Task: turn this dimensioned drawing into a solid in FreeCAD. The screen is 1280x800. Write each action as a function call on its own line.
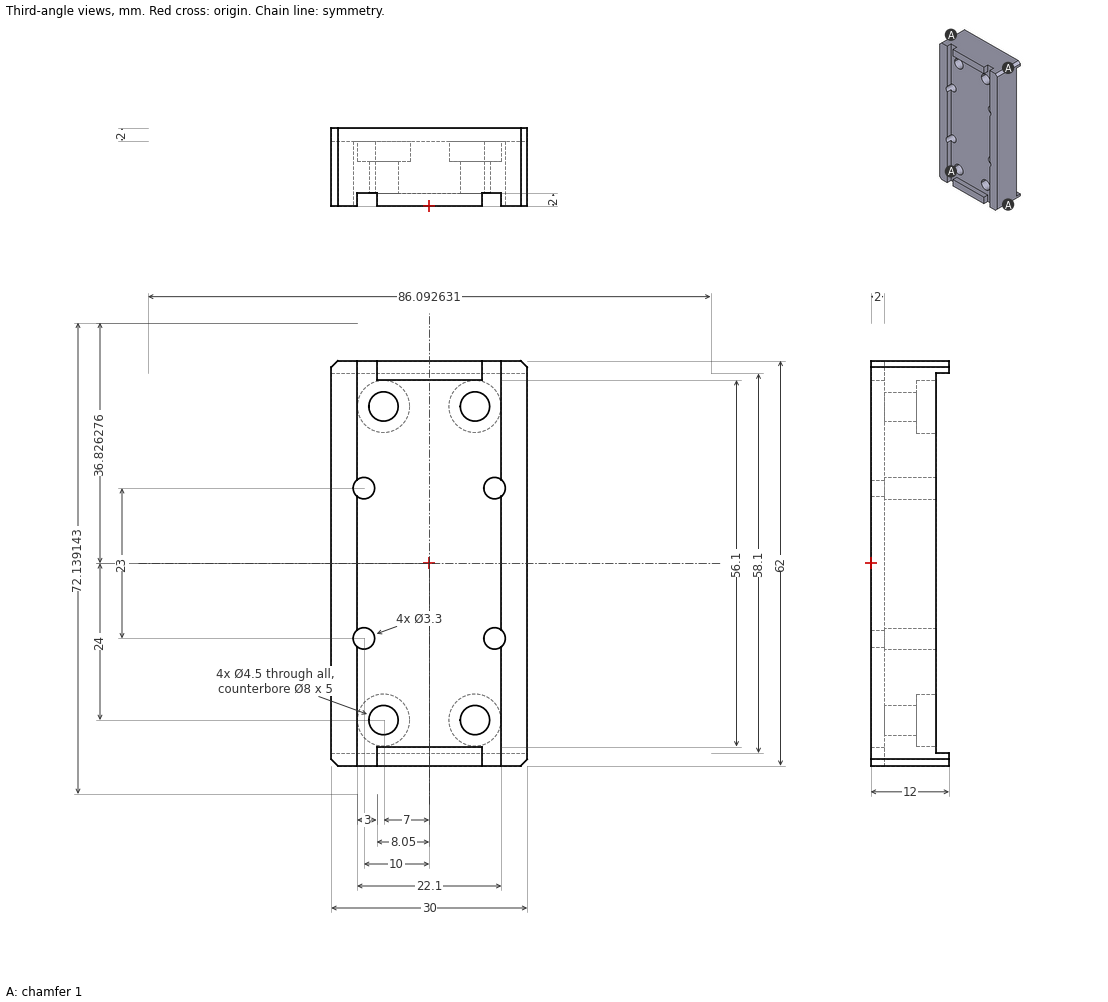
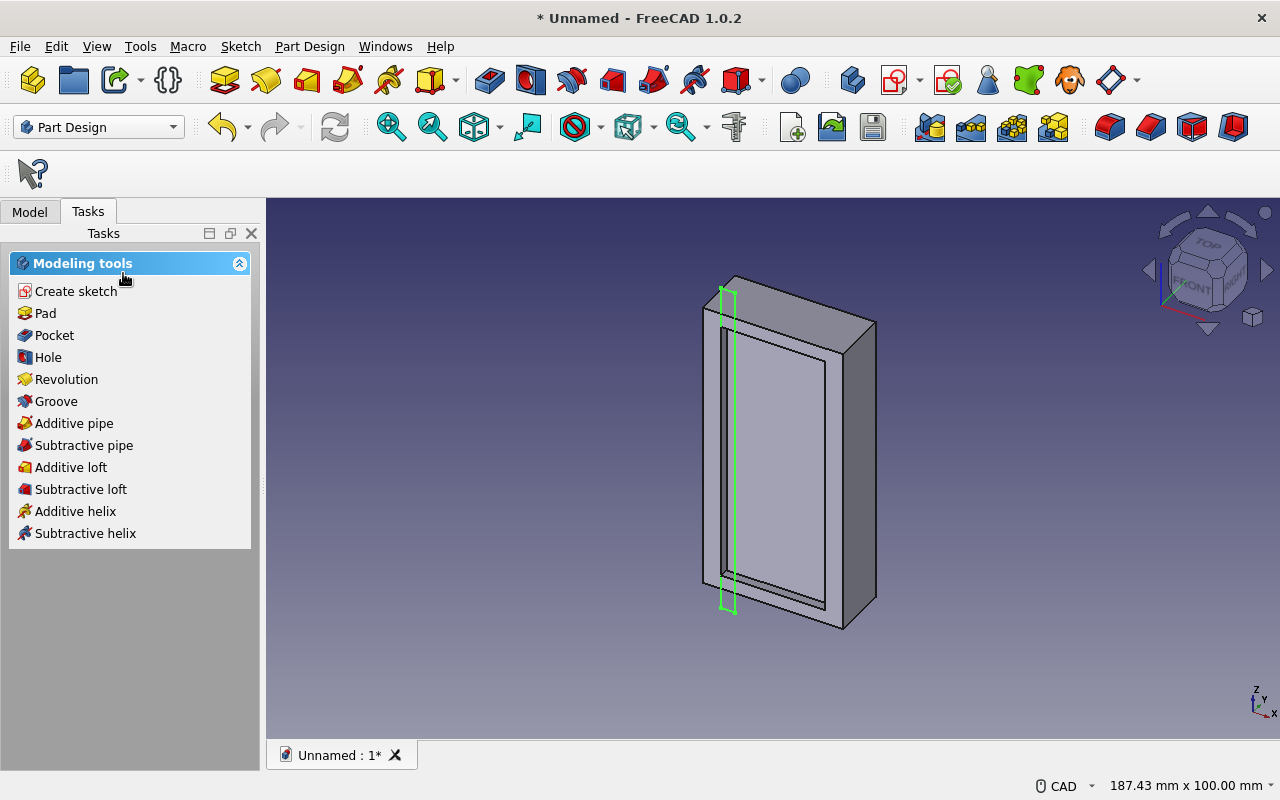
click(490, 80)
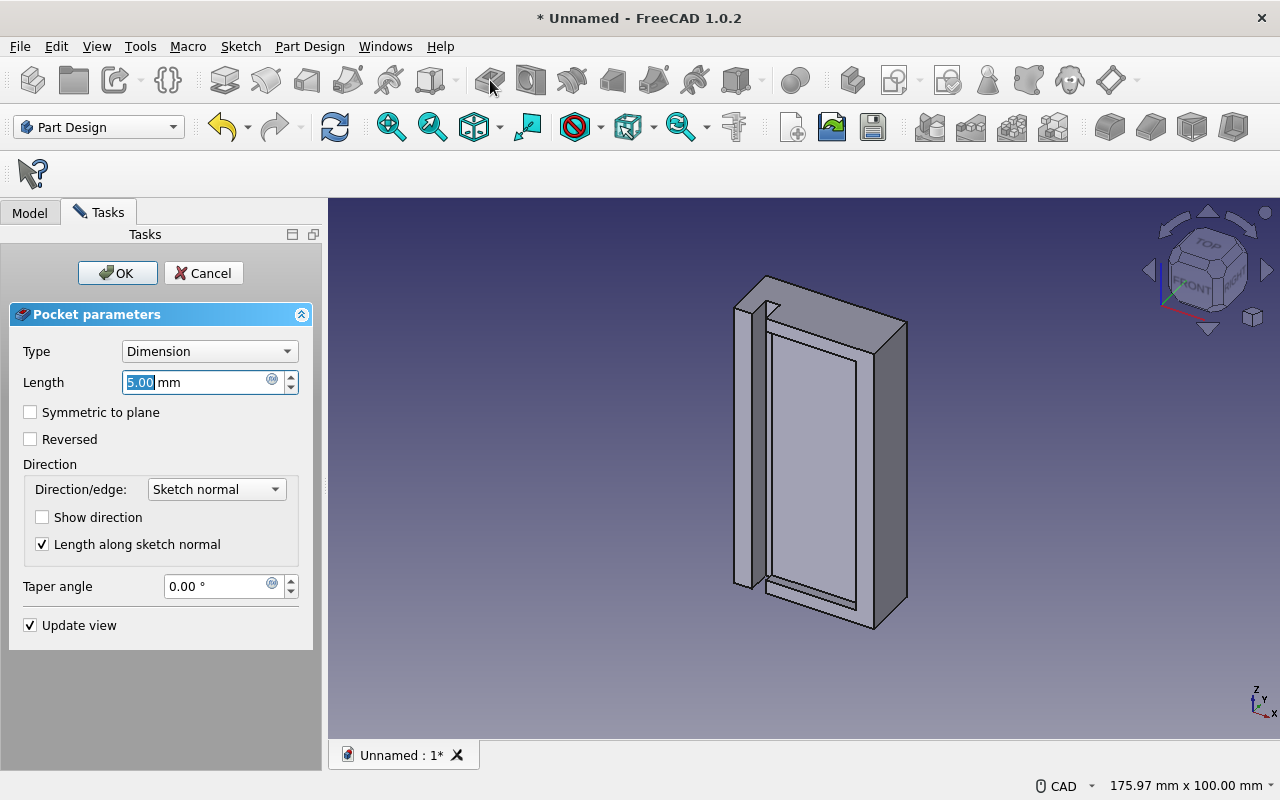
text(2)
key(Tab)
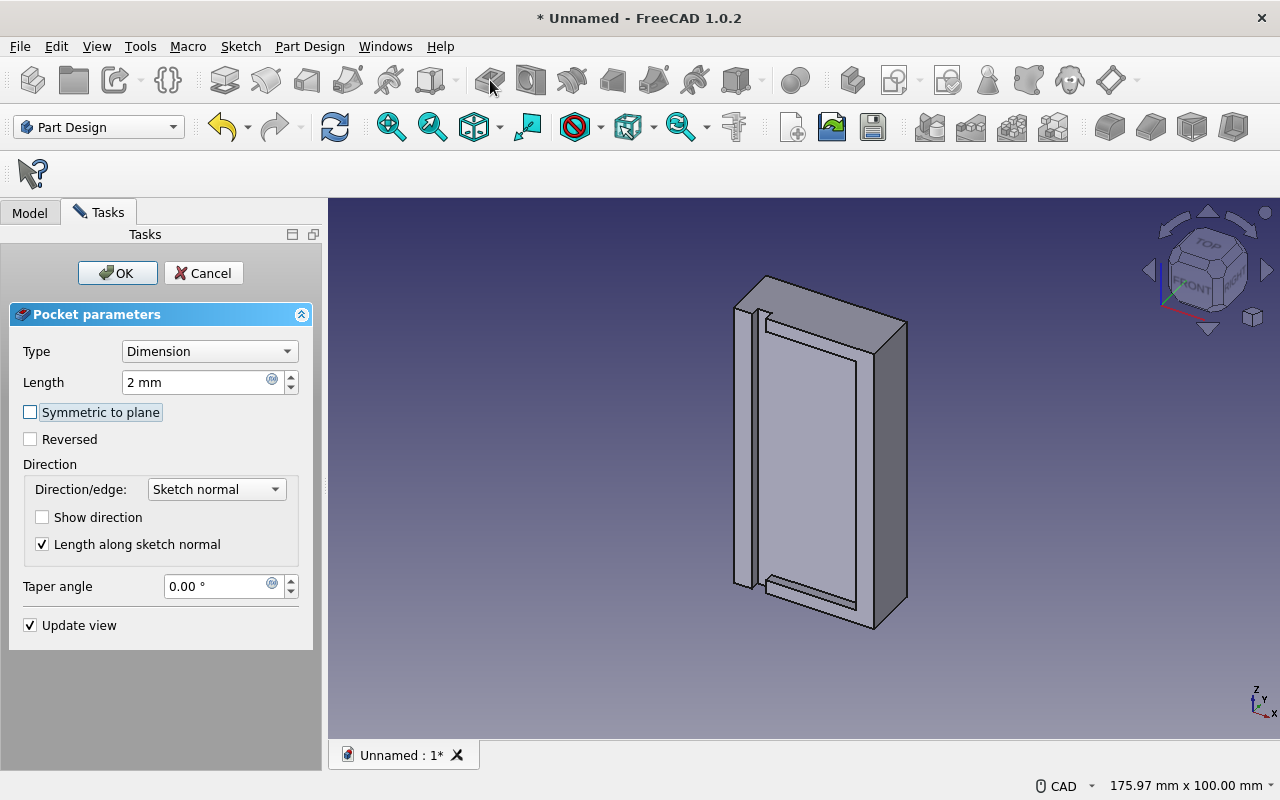
click(118, 273)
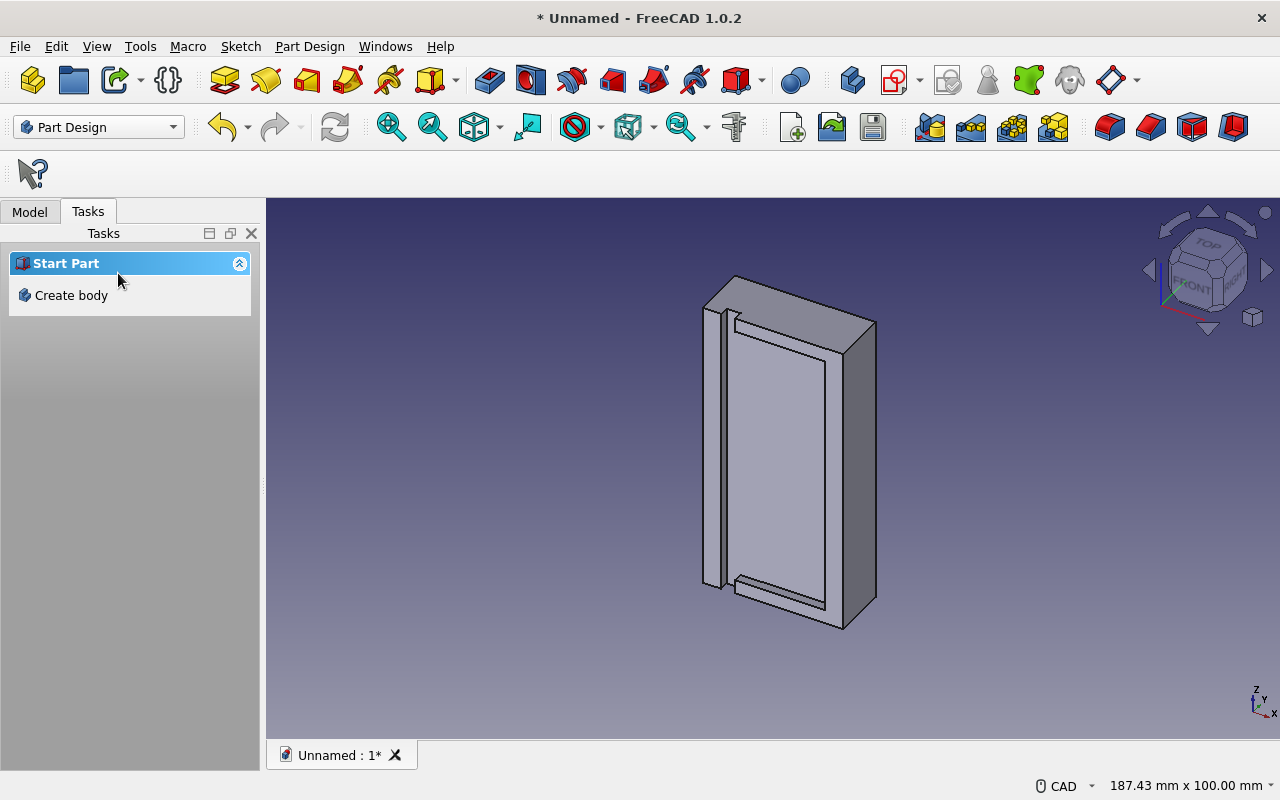
click(30, 212)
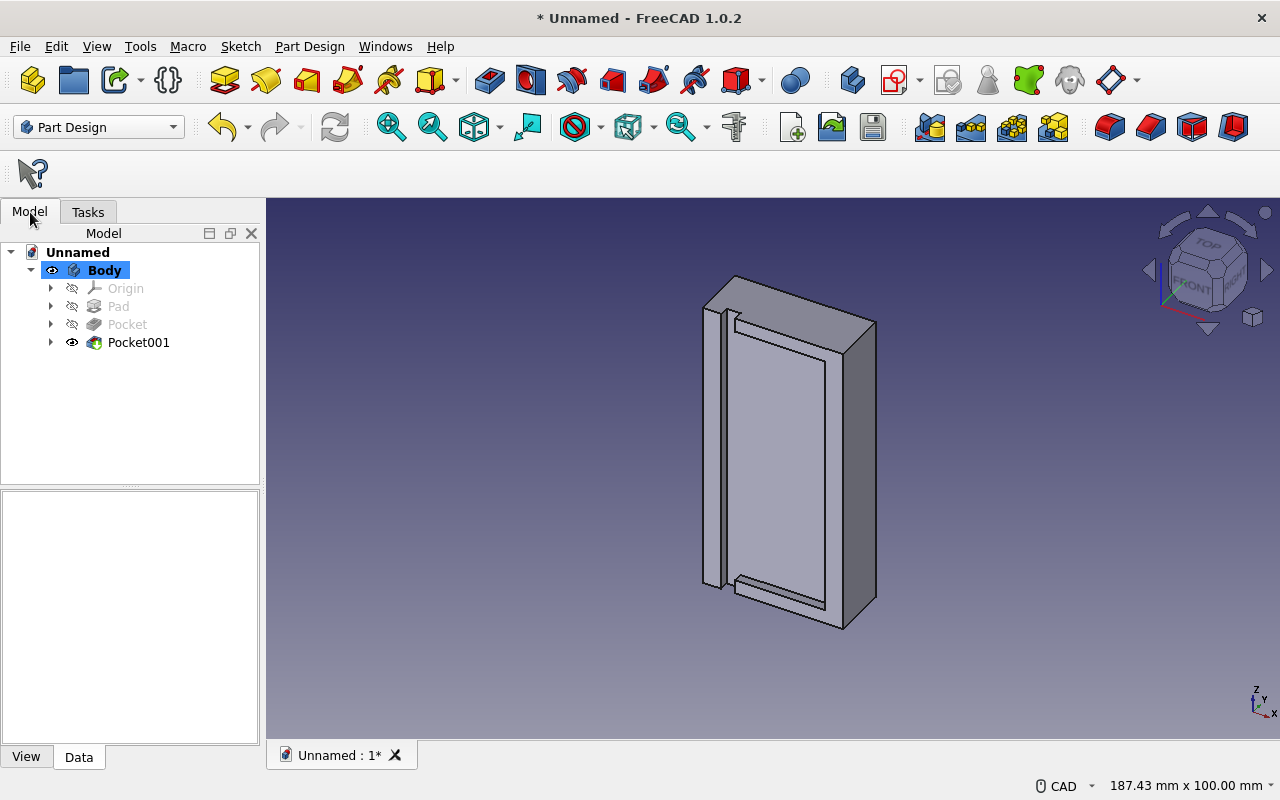
click(117, 342)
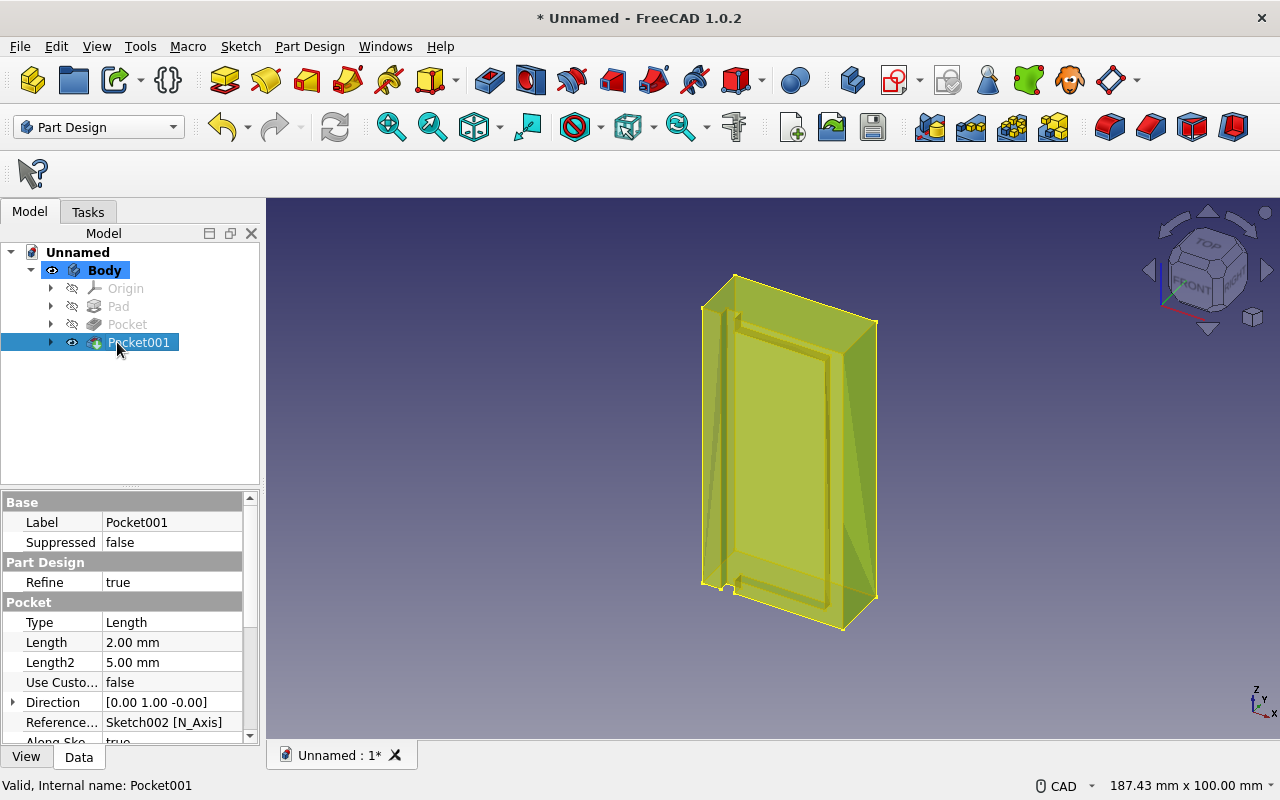
click(930, 128)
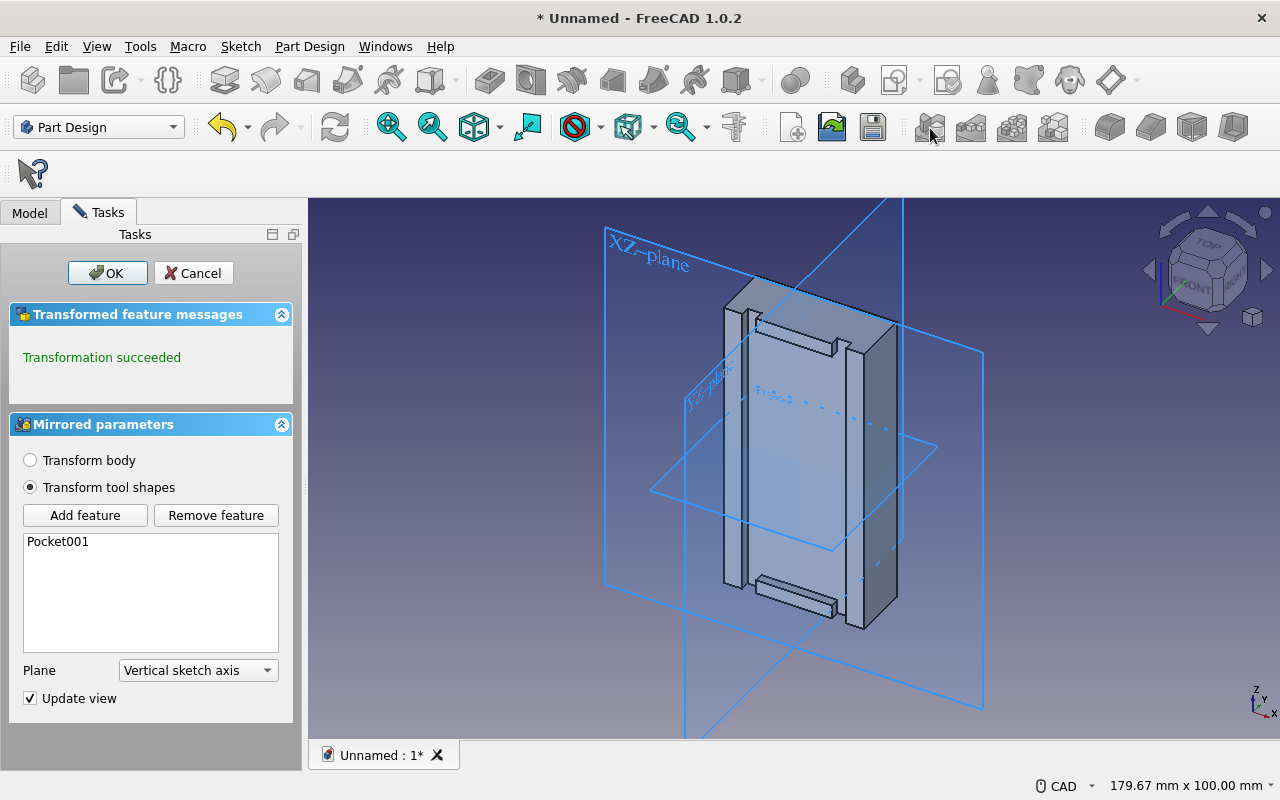
click(199, 670)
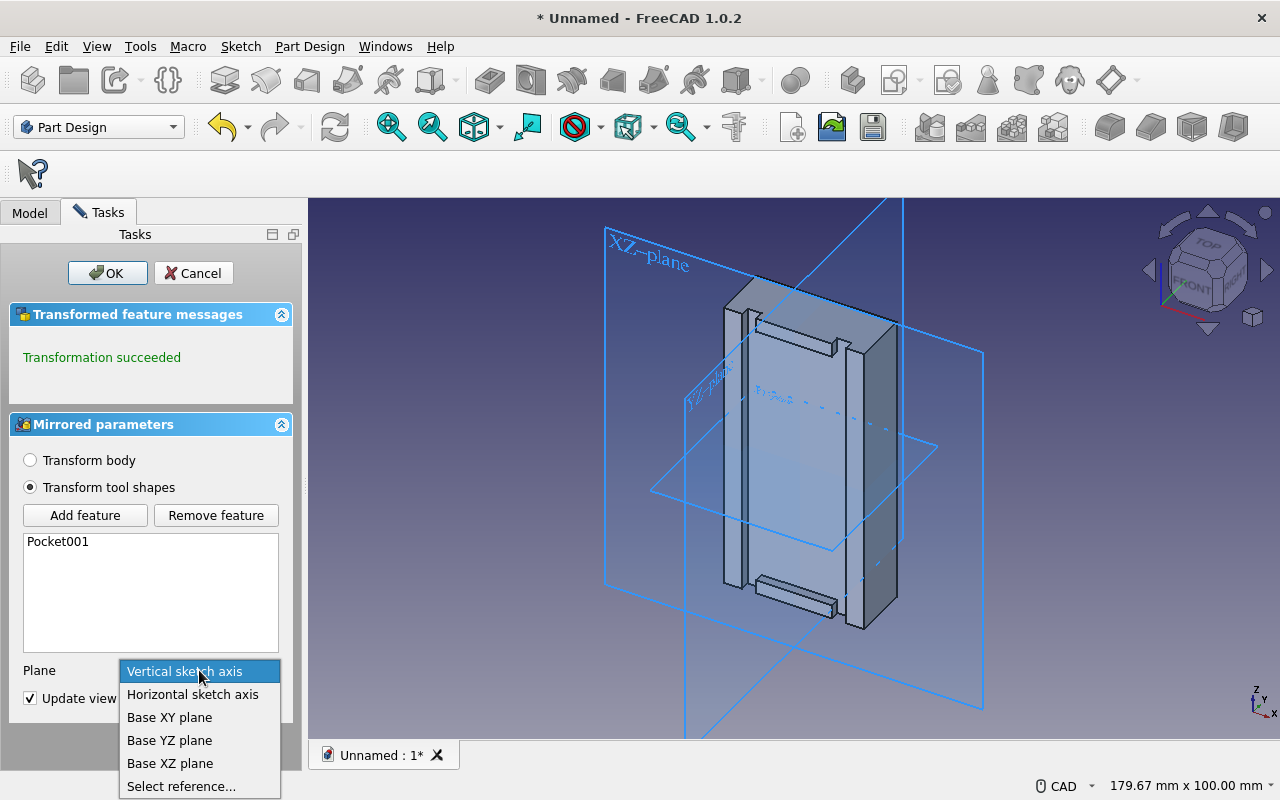
click(198, 740)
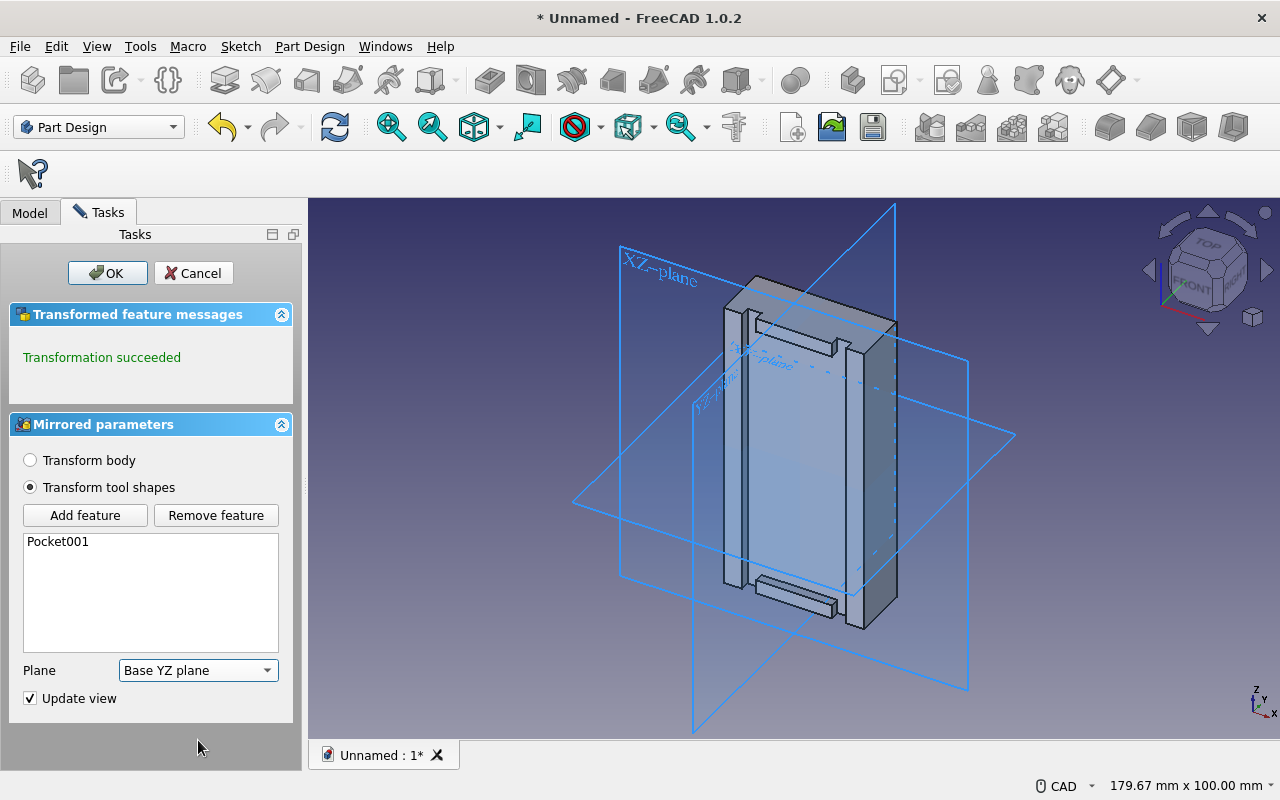
click(108, 273)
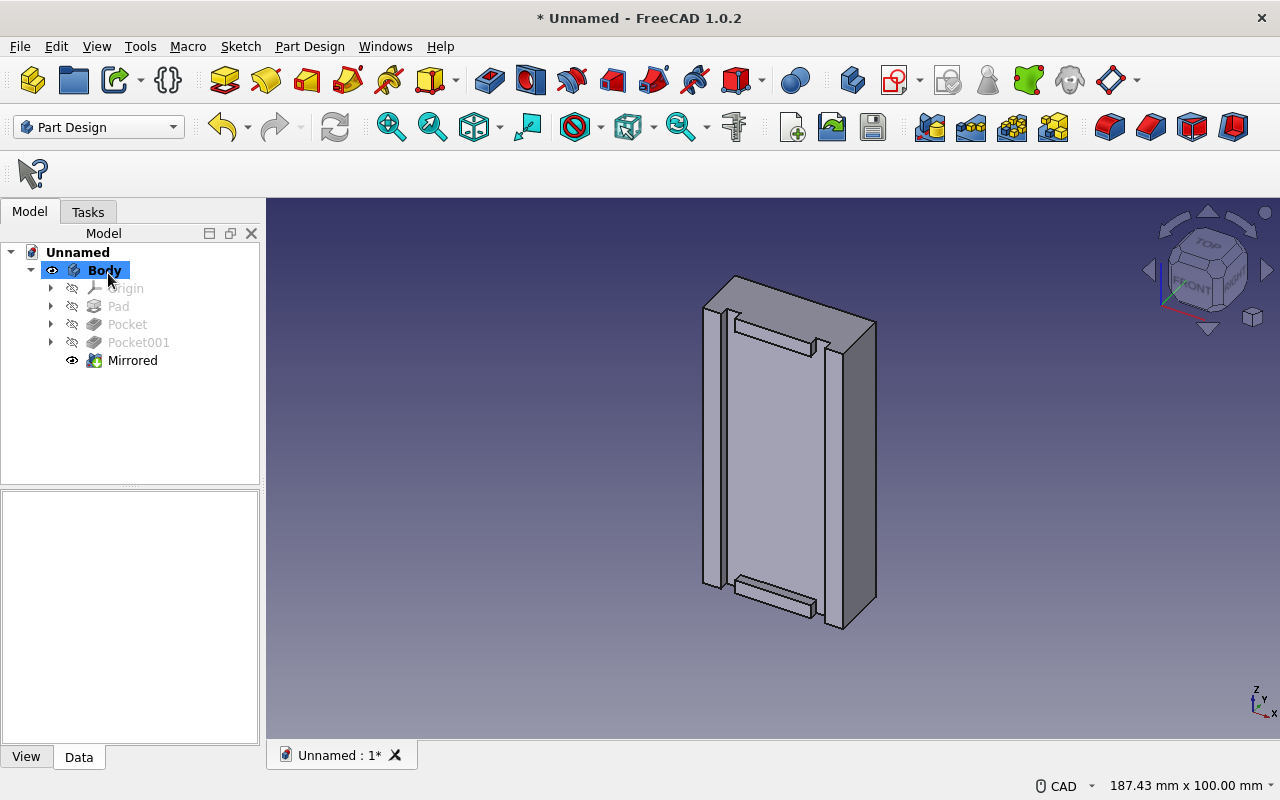
key(4)